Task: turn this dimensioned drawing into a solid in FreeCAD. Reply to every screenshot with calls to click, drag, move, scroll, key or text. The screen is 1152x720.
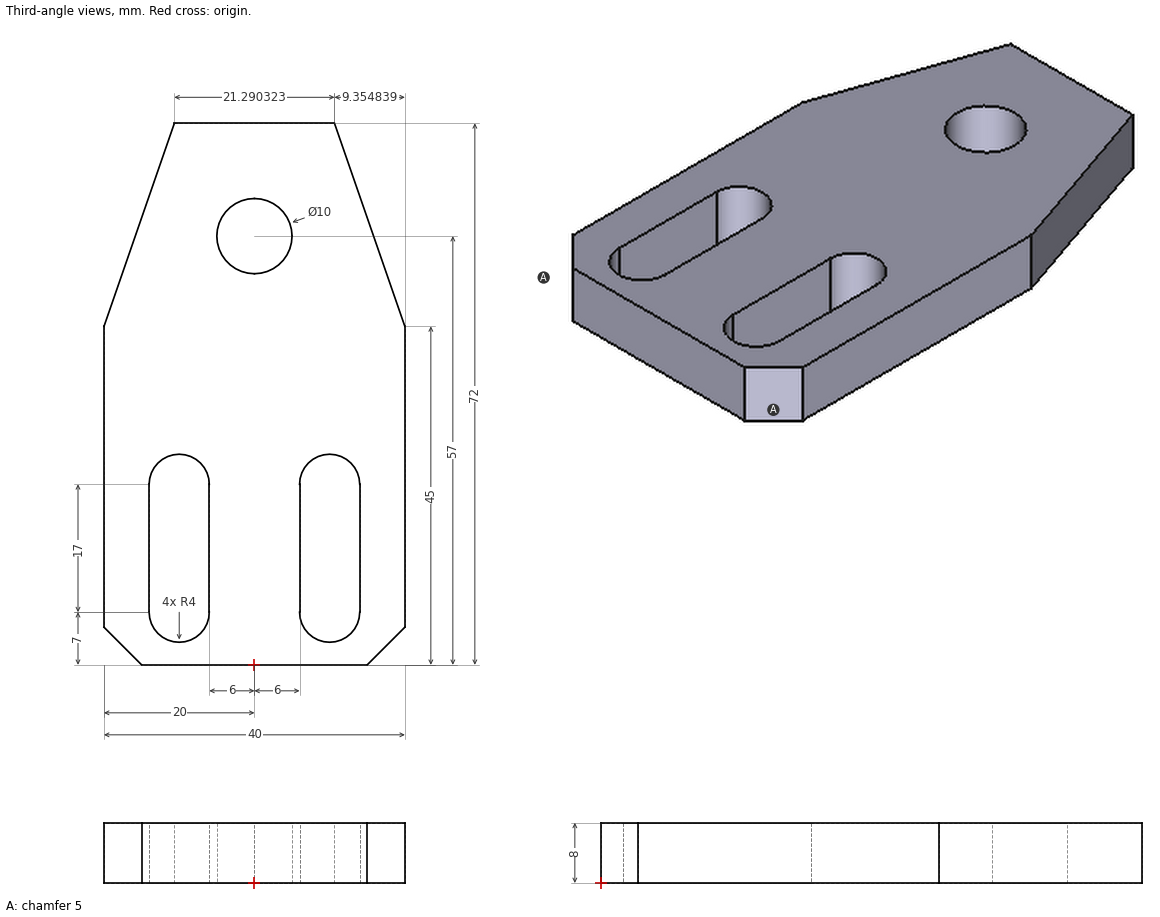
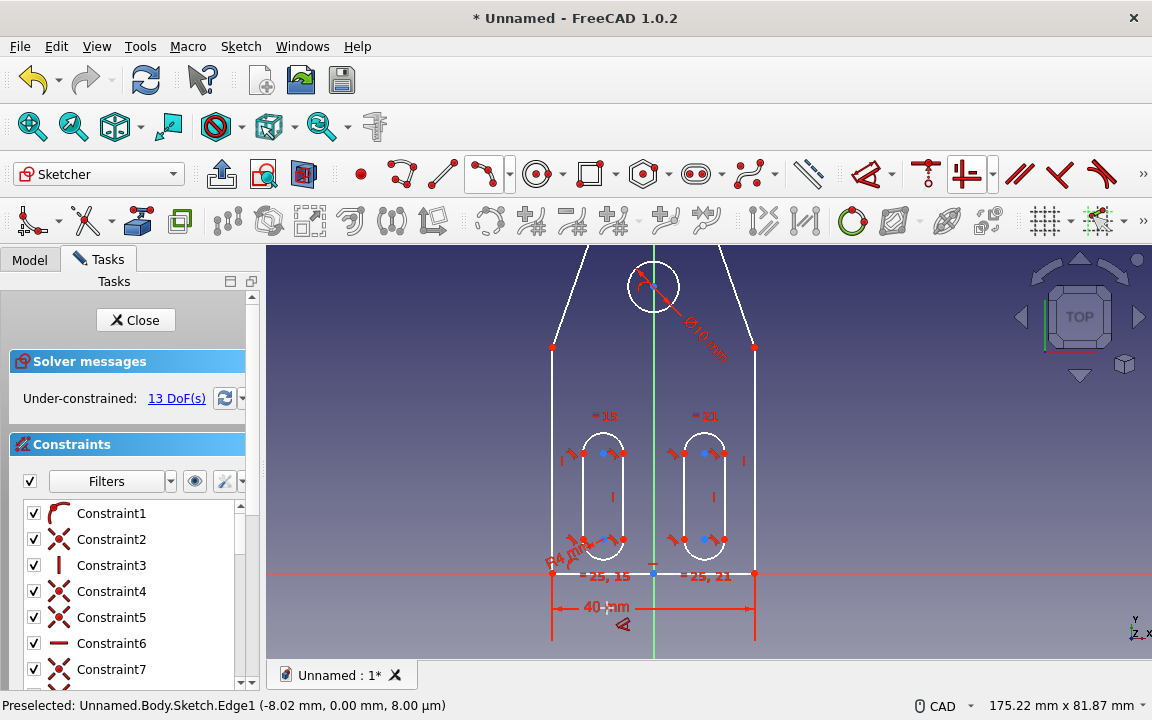
click(755, 506)
click(789, 461)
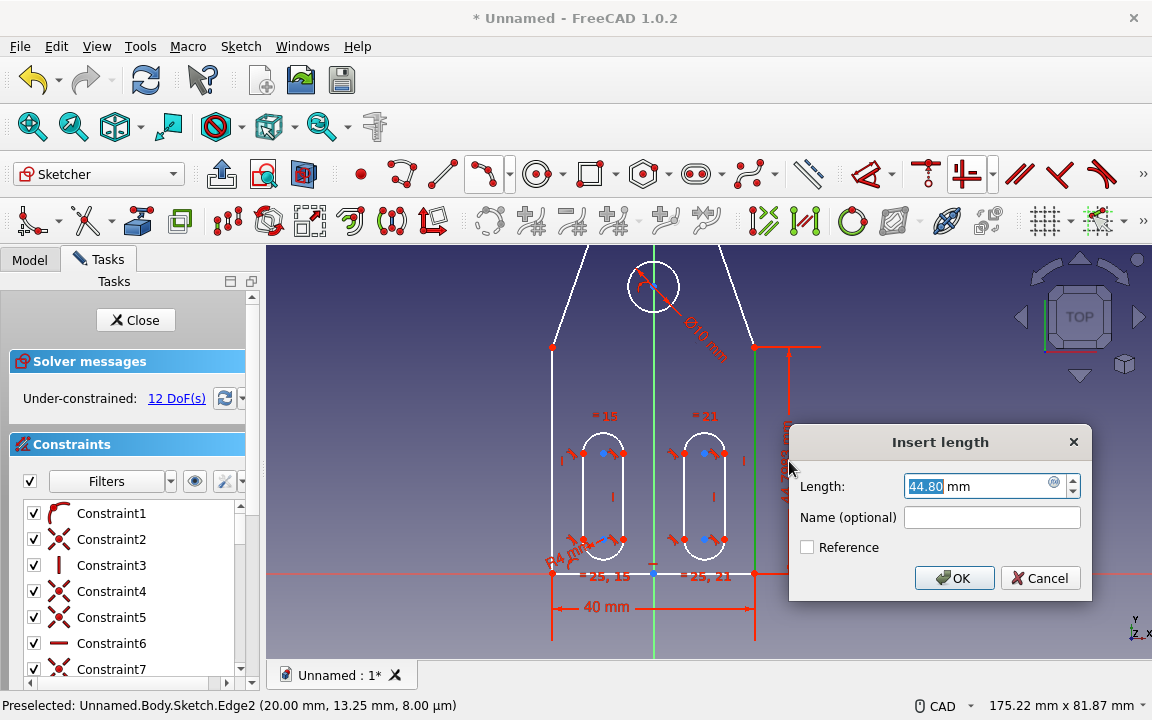
text(45)
key(Return)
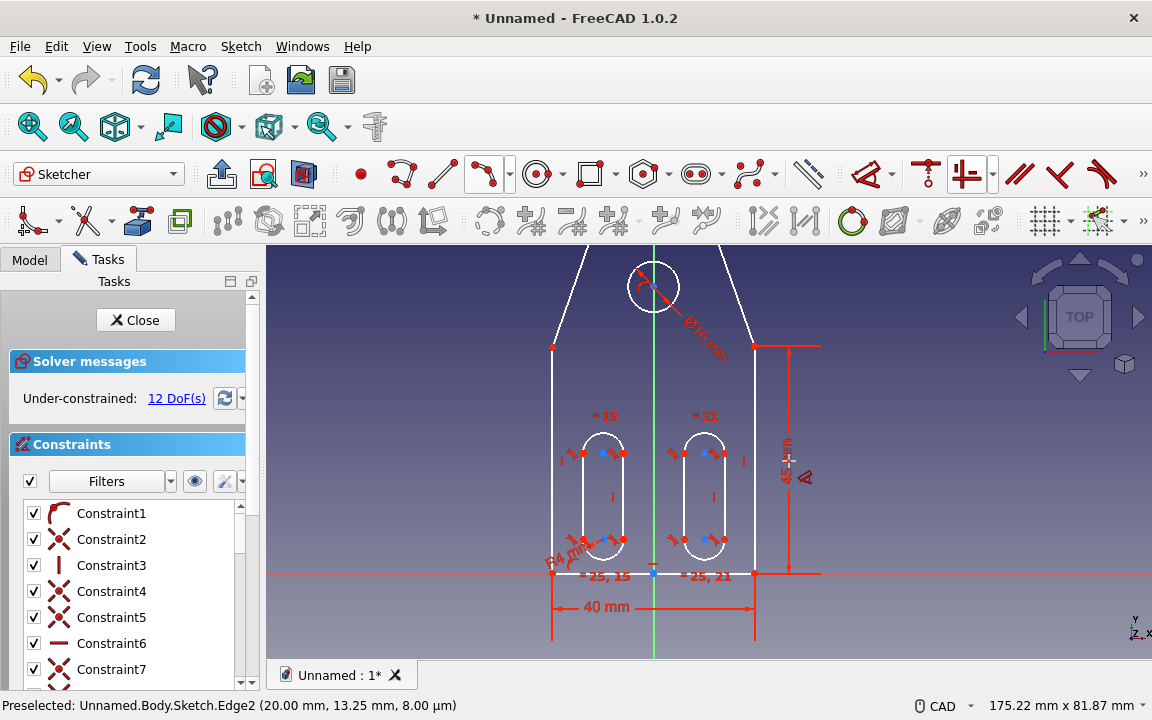
click(552, 415)
click(518, 461)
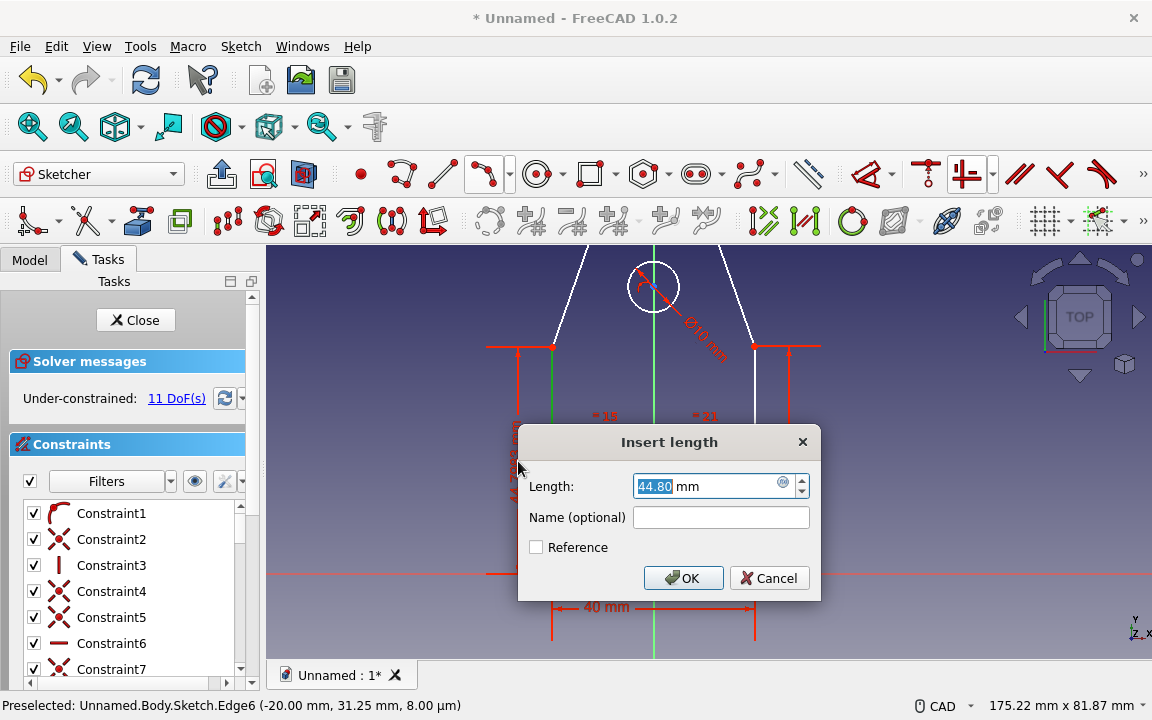
text(45)
key(Return)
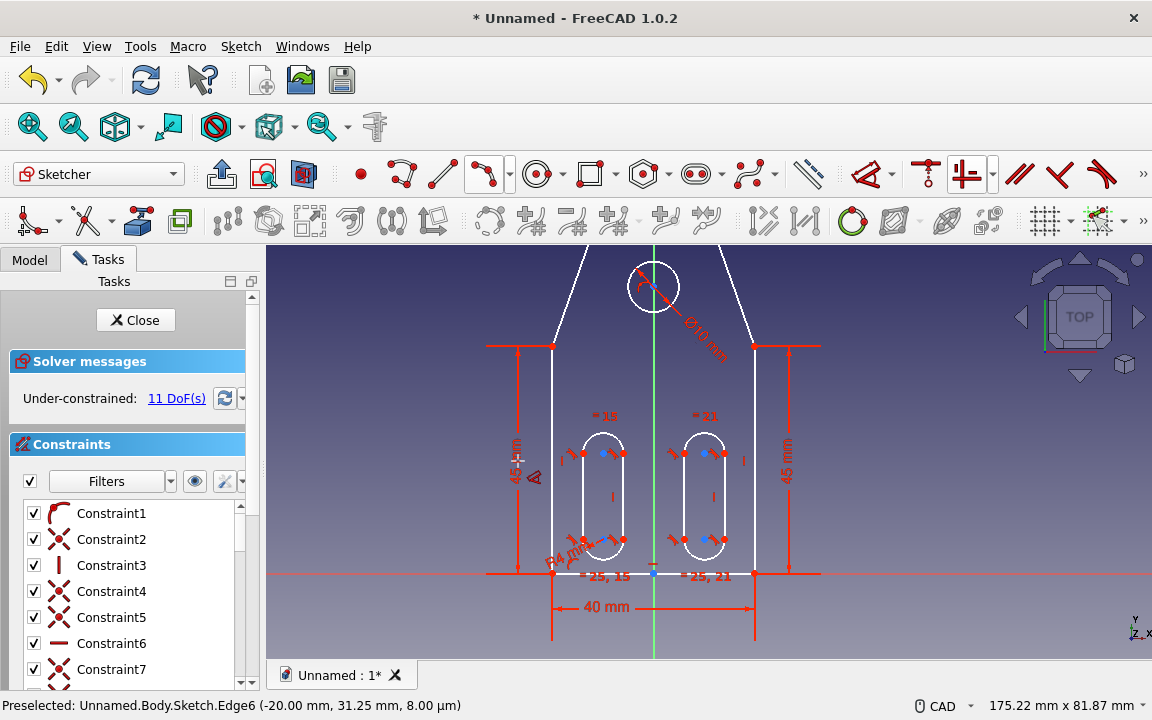
click(583, 514)
click(525, 496)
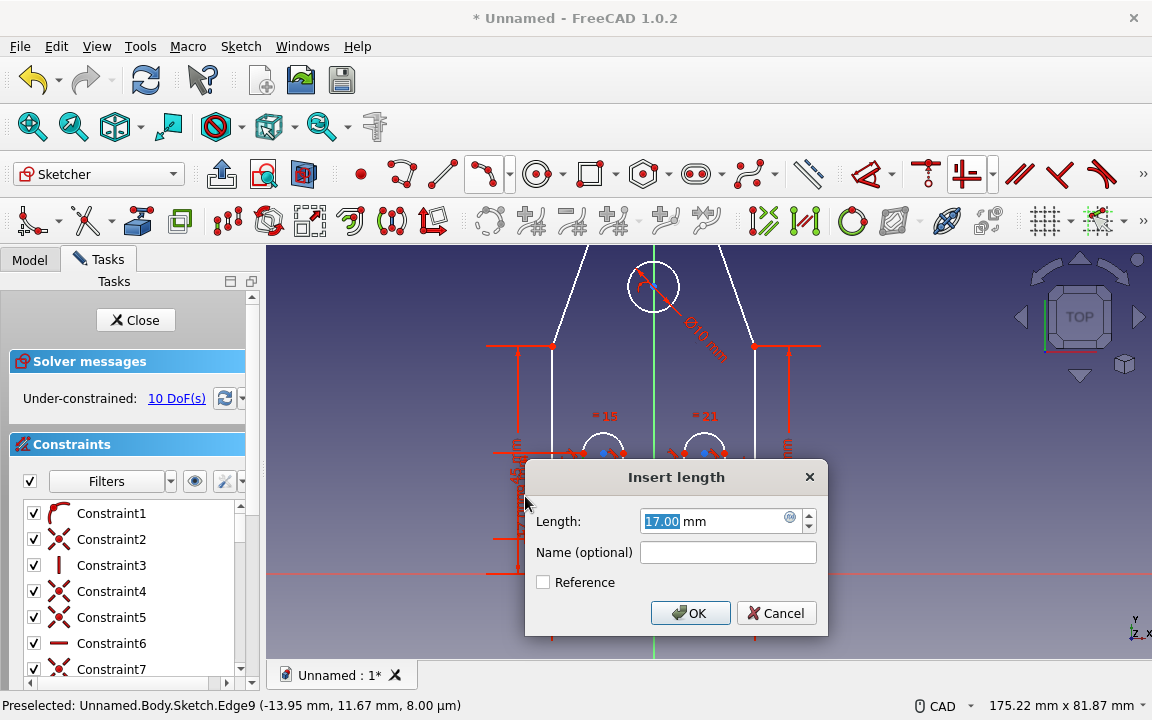
text(17)
key(Return)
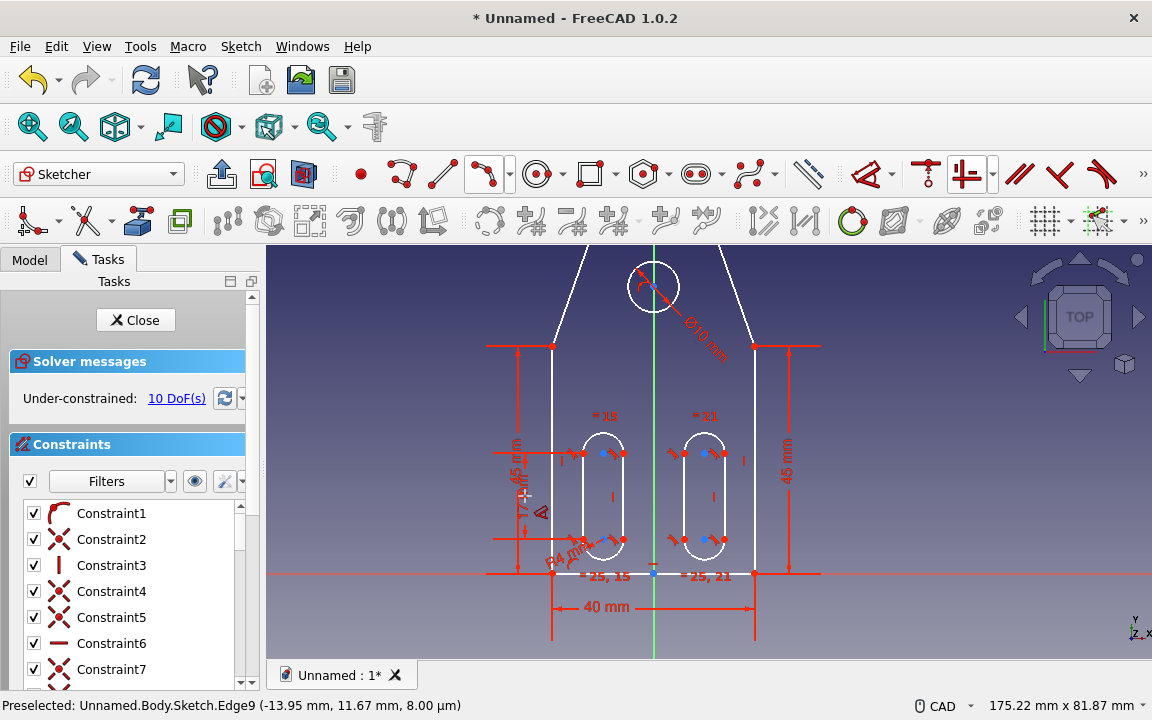
click(684, 514)
click(602, 496)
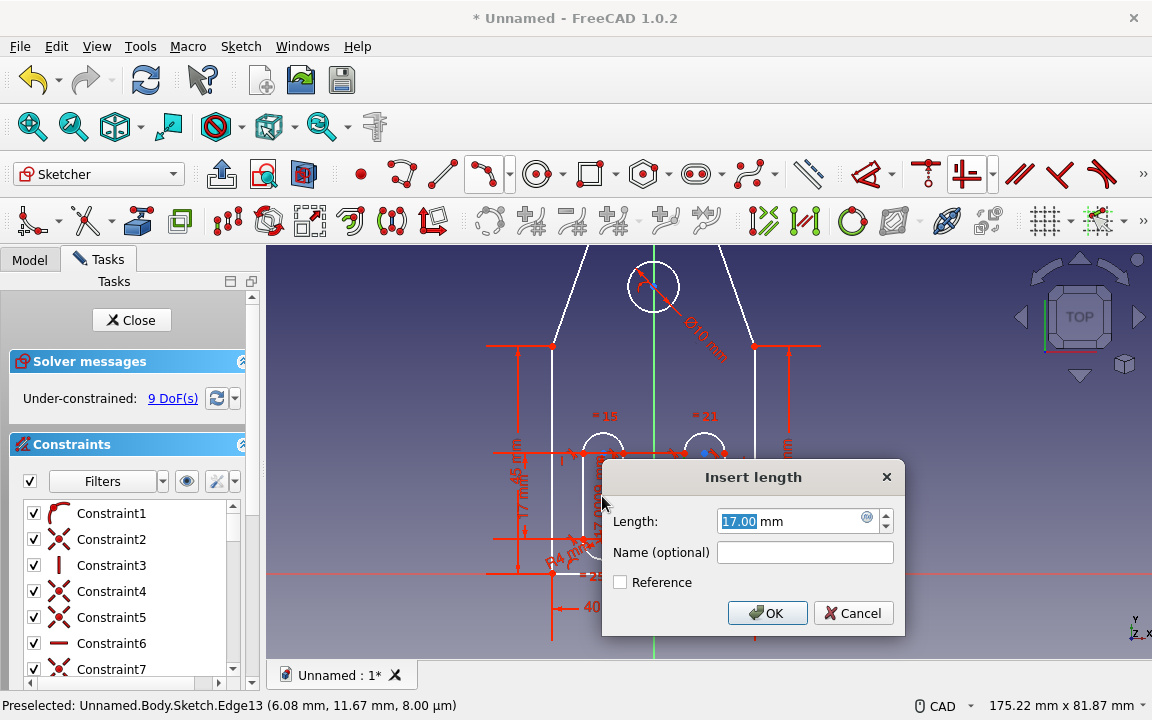
text(17)
key(Return)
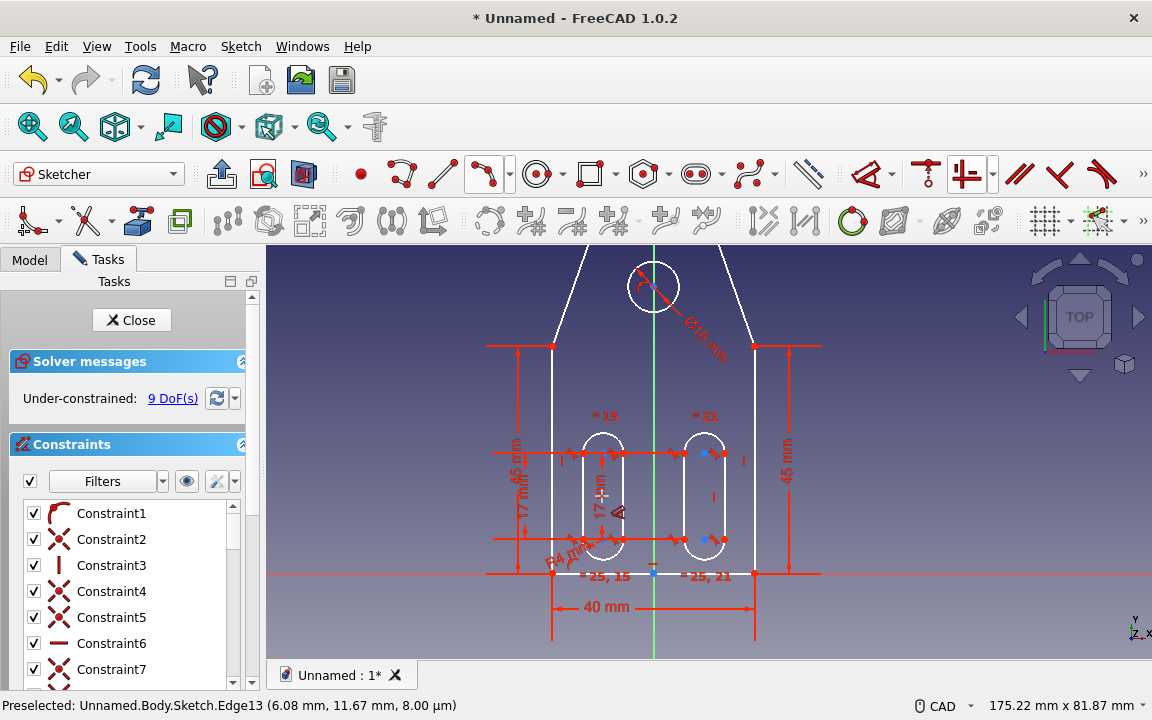
click(583, 539)
click(736, 557)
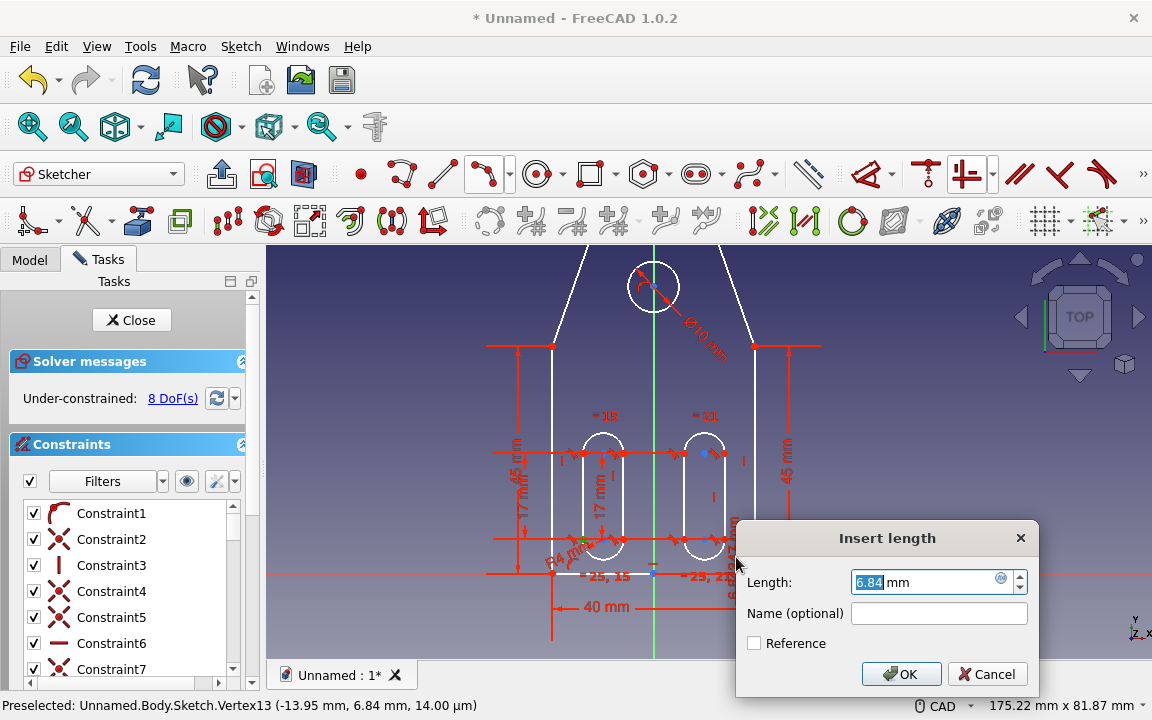
text(7)
key(Return)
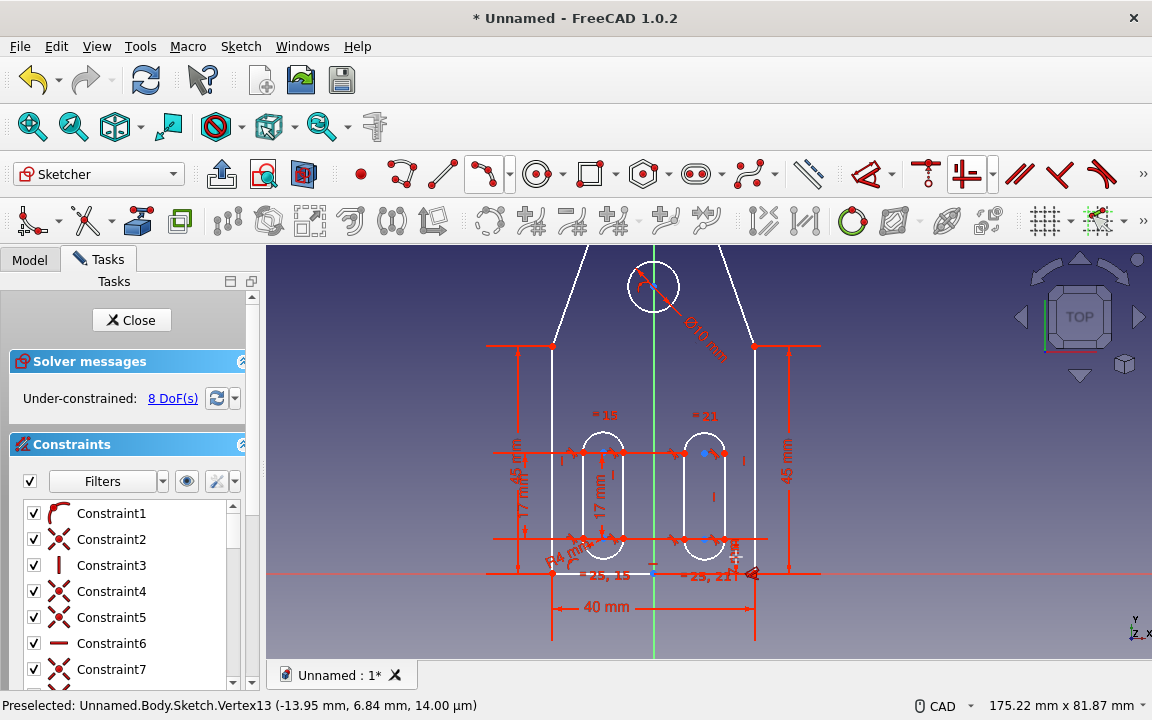
scroll(623, 539, up, 2)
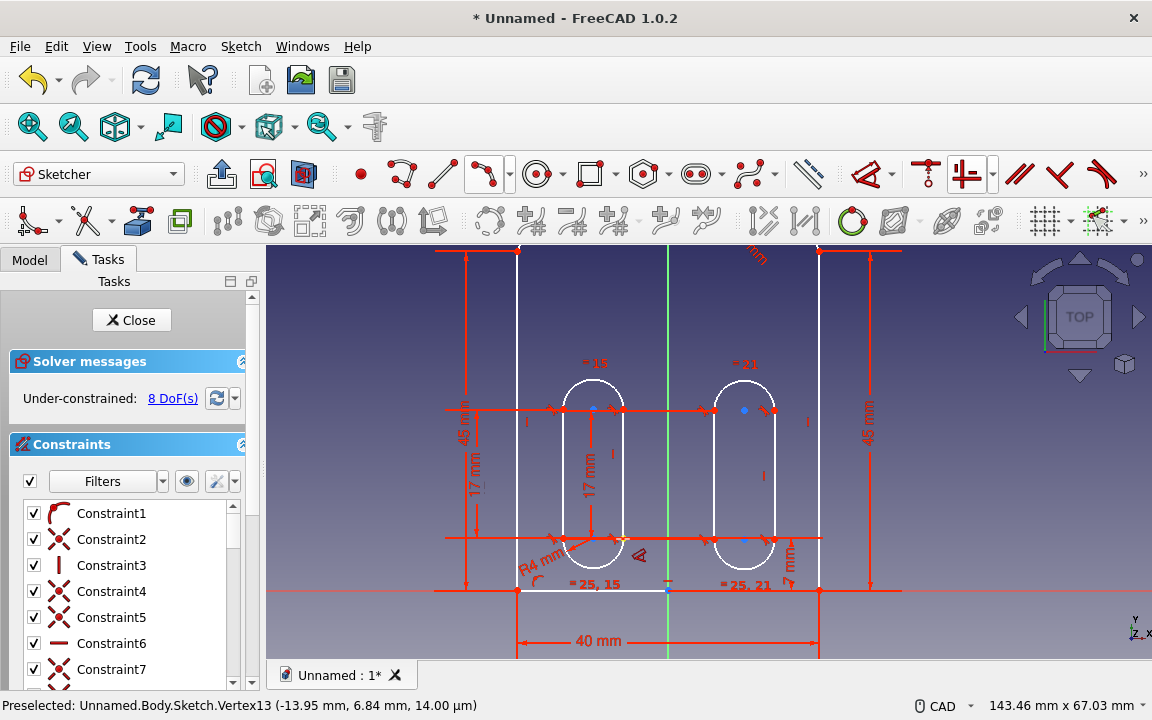
click(623, 538)
click(646, 504)